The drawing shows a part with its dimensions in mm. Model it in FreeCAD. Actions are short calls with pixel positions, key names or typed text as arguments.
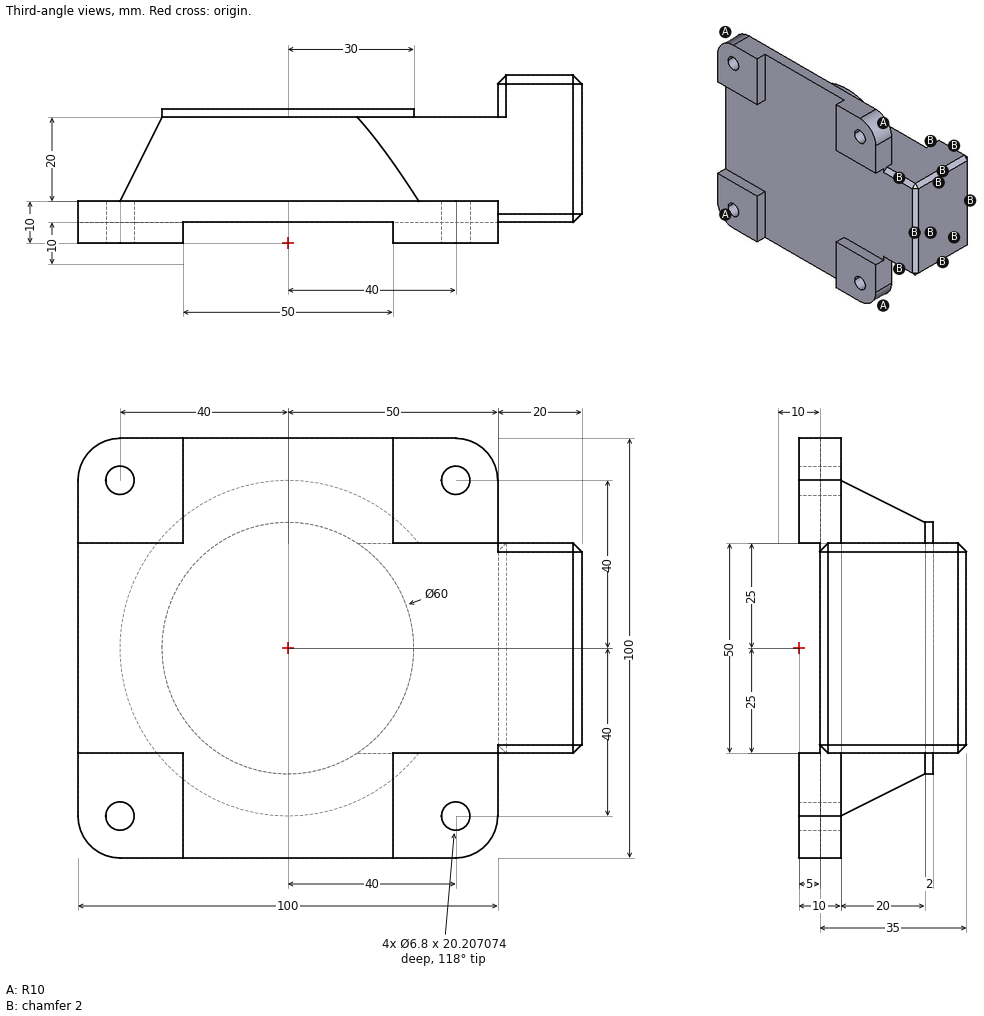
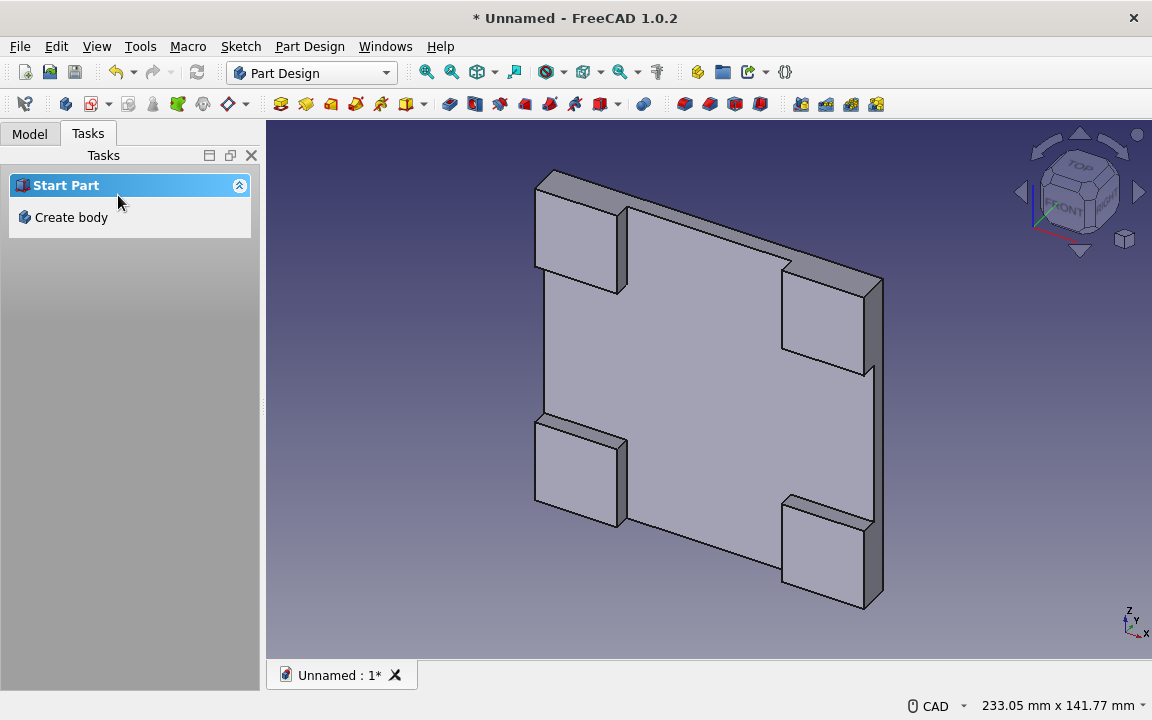
click(874, 287)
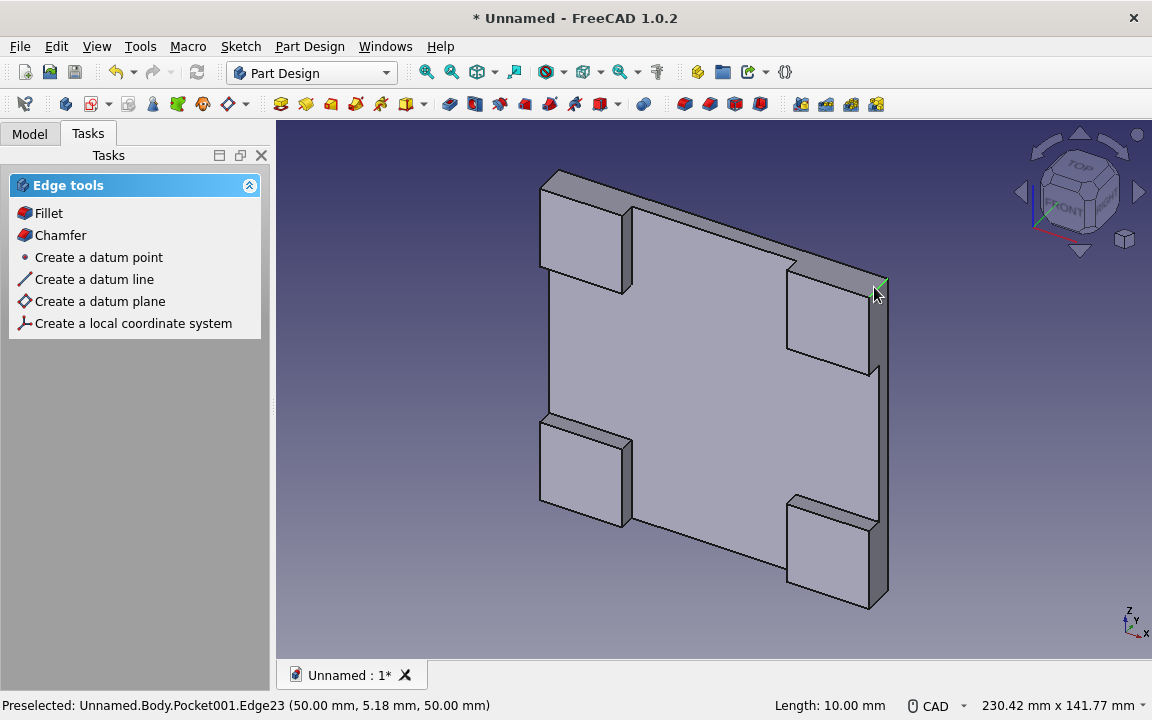
key(0)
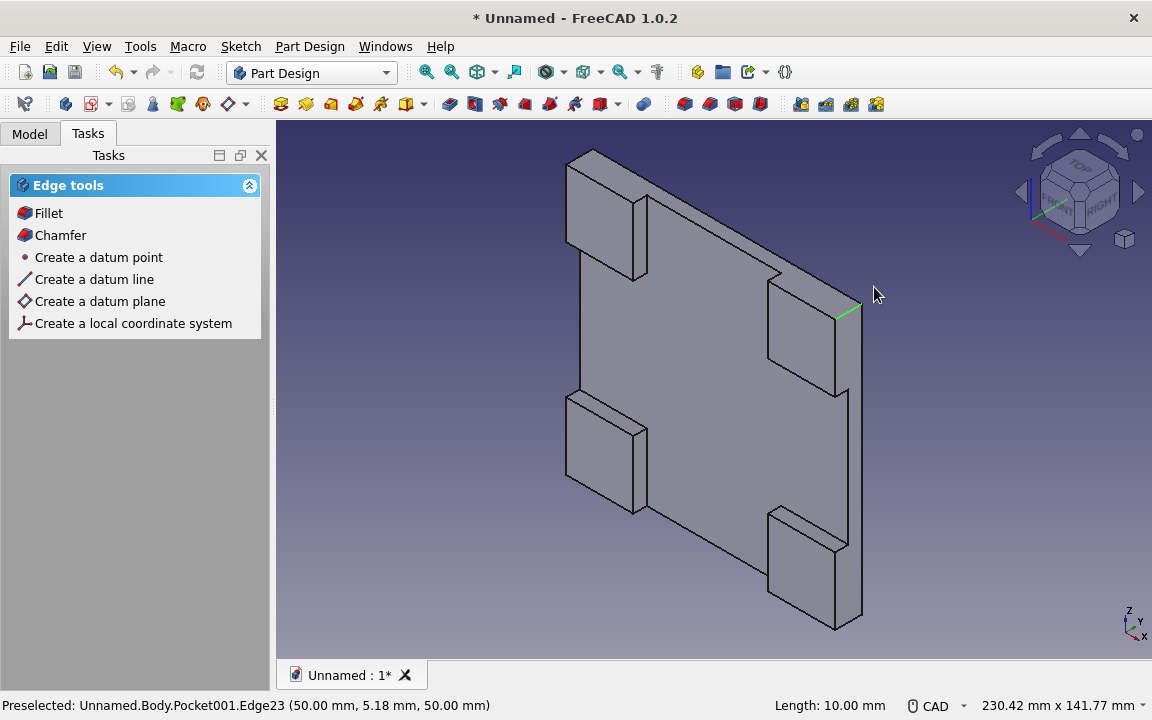
key(2)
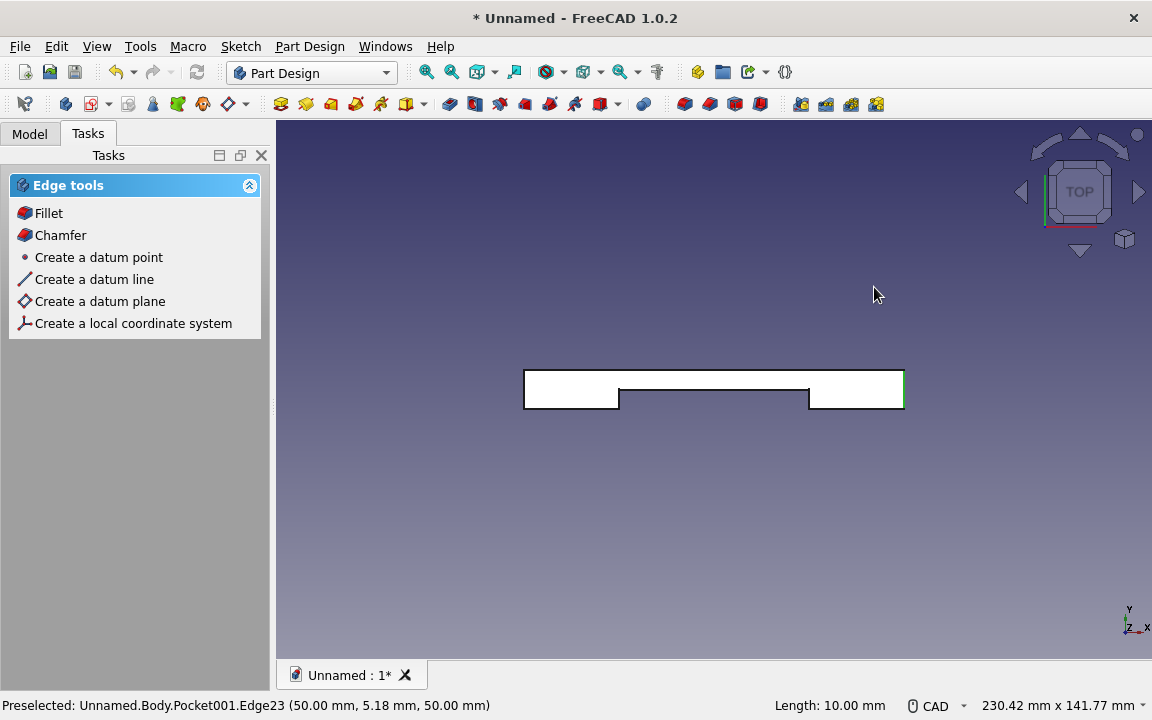
key(v)
key(f)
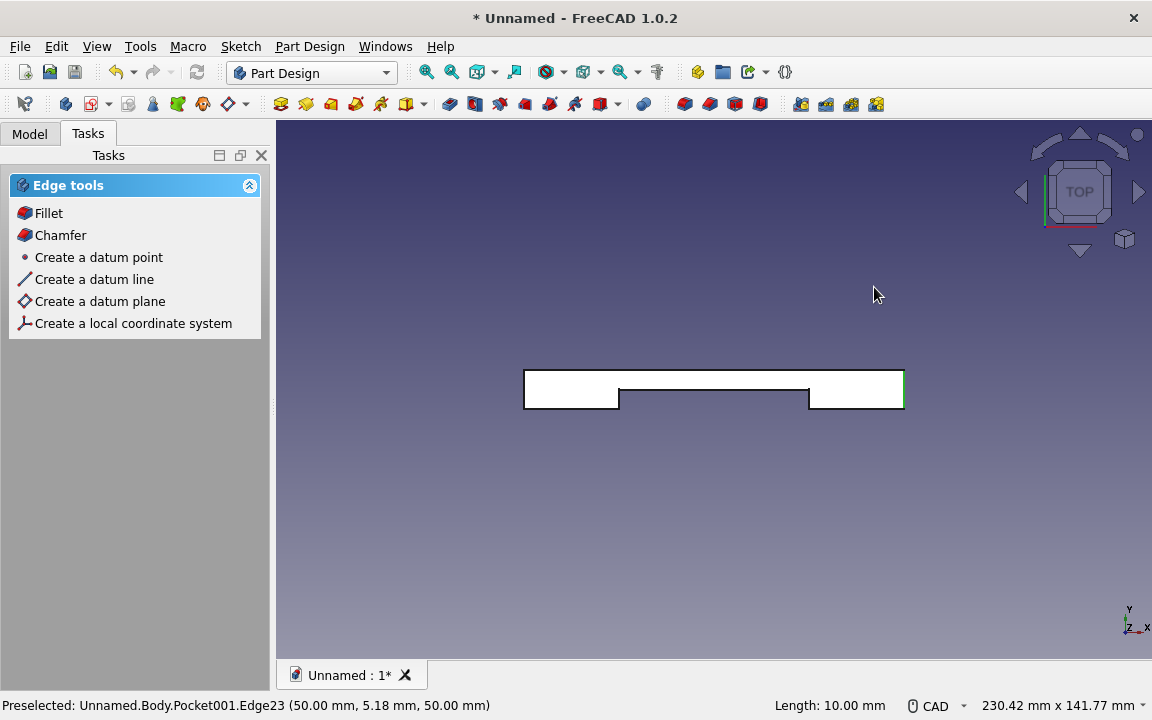
click(524, 388, ctrl)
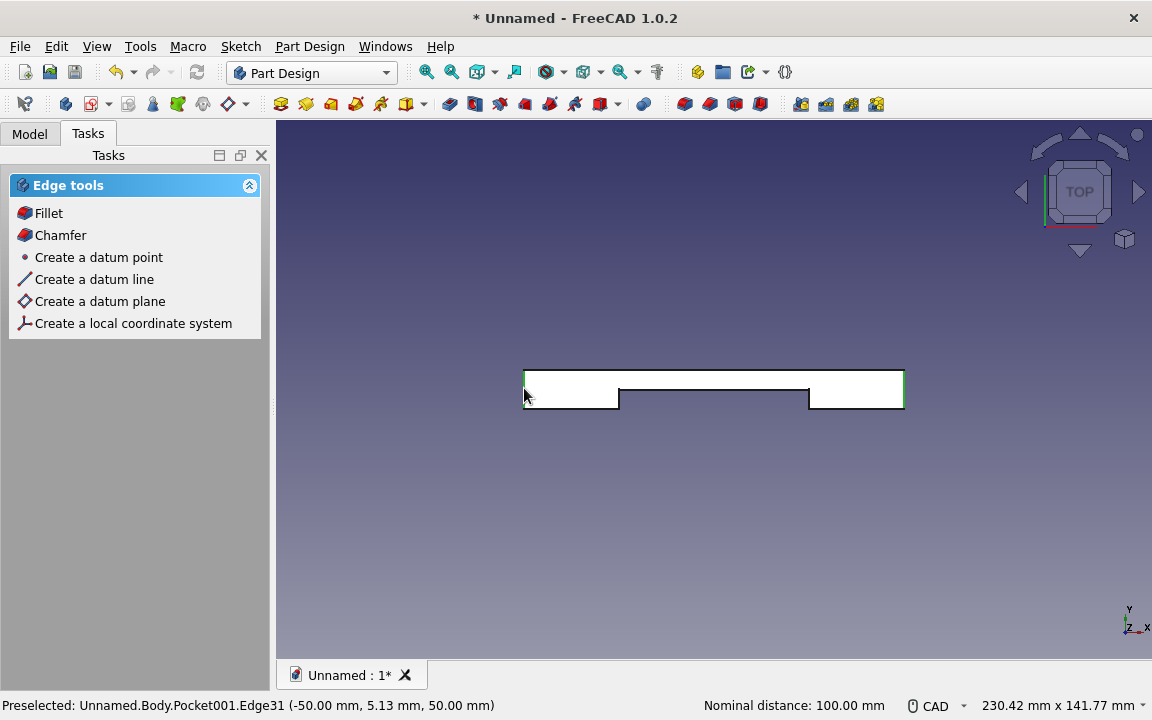
key(1)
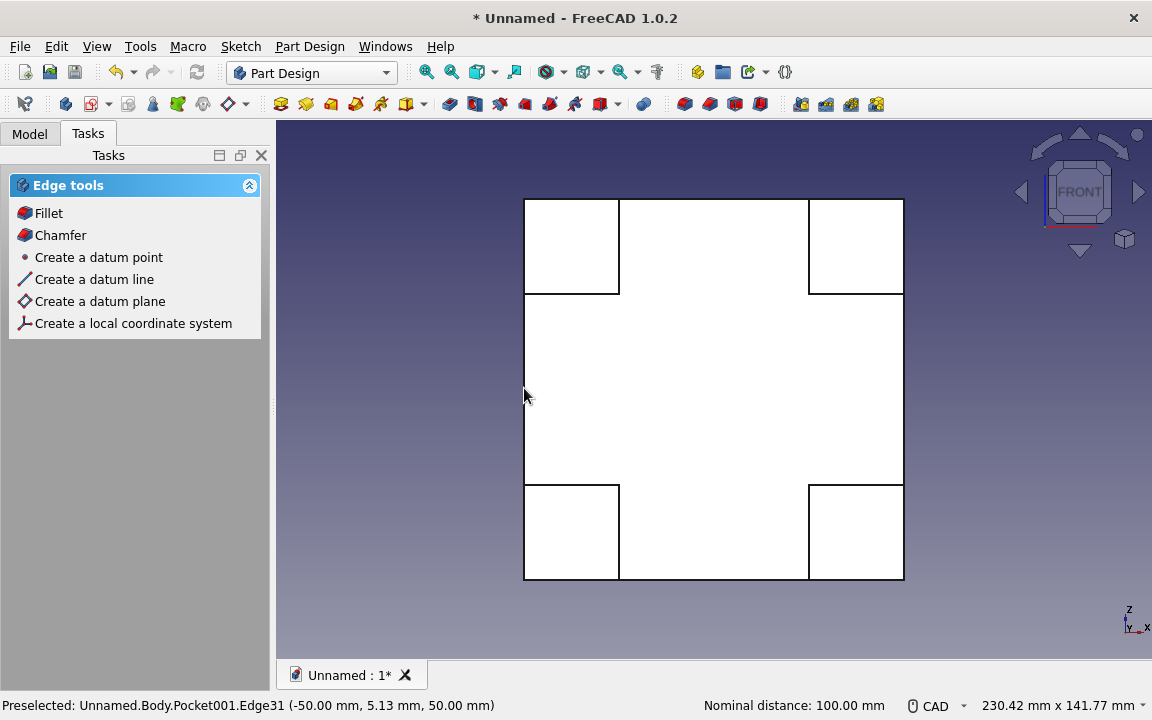
key(3)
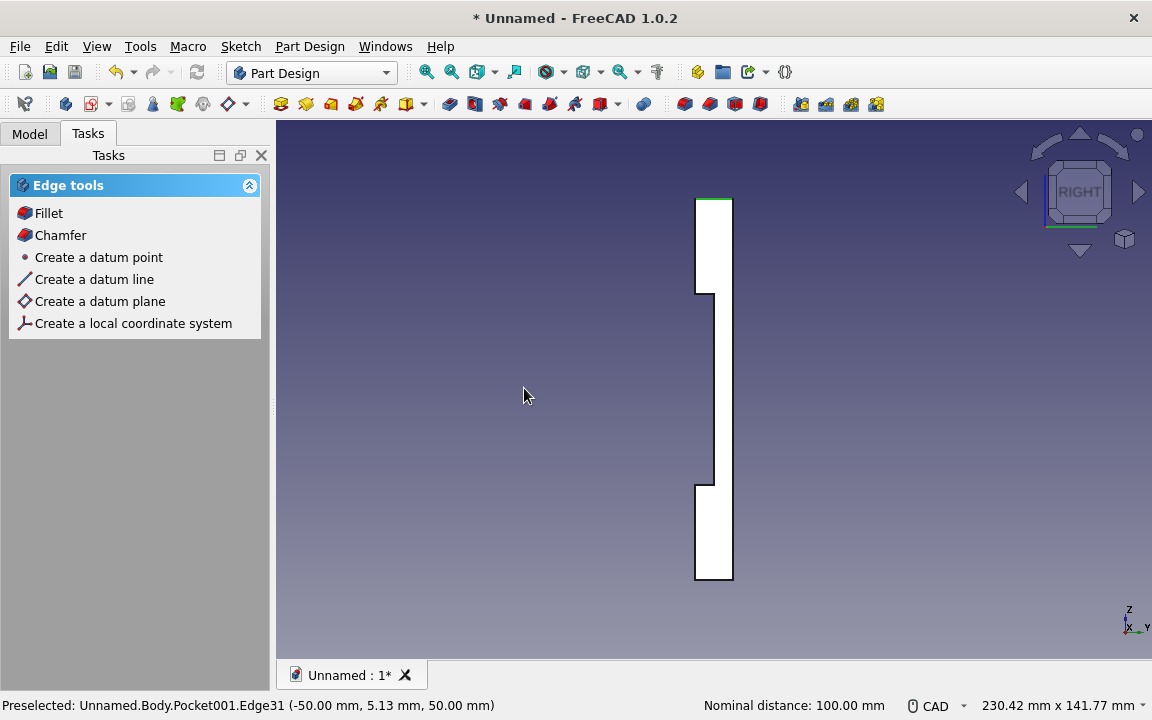
click(714, 579, ctrl)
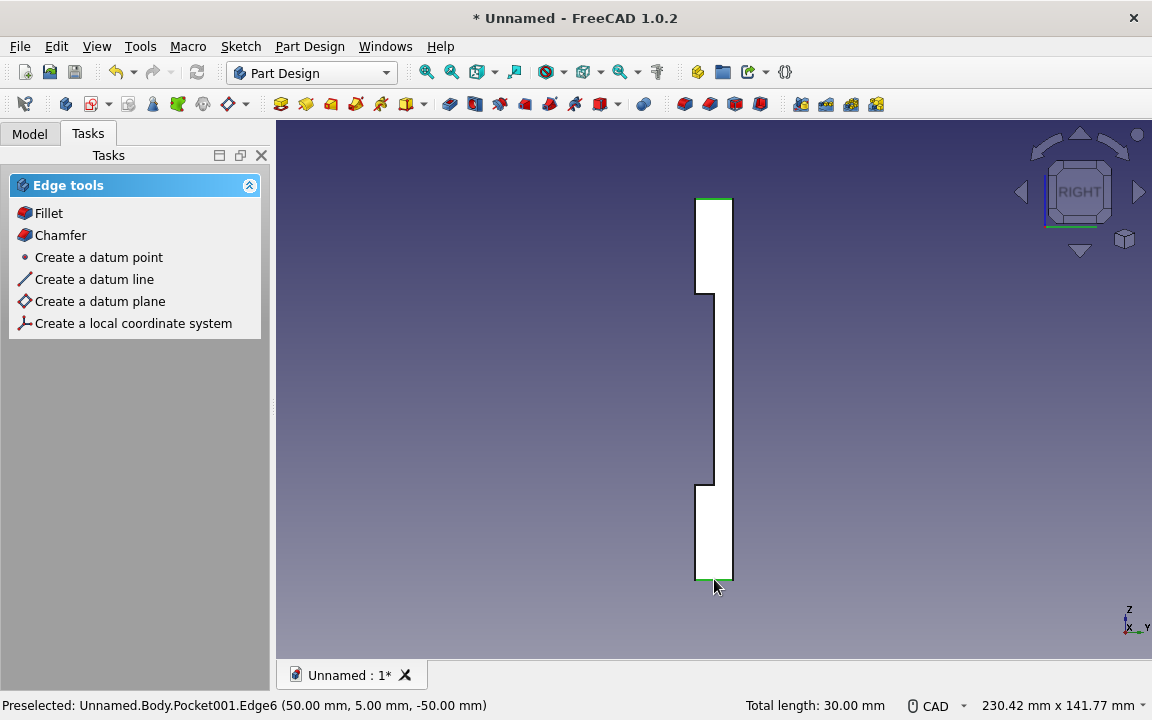
key(5)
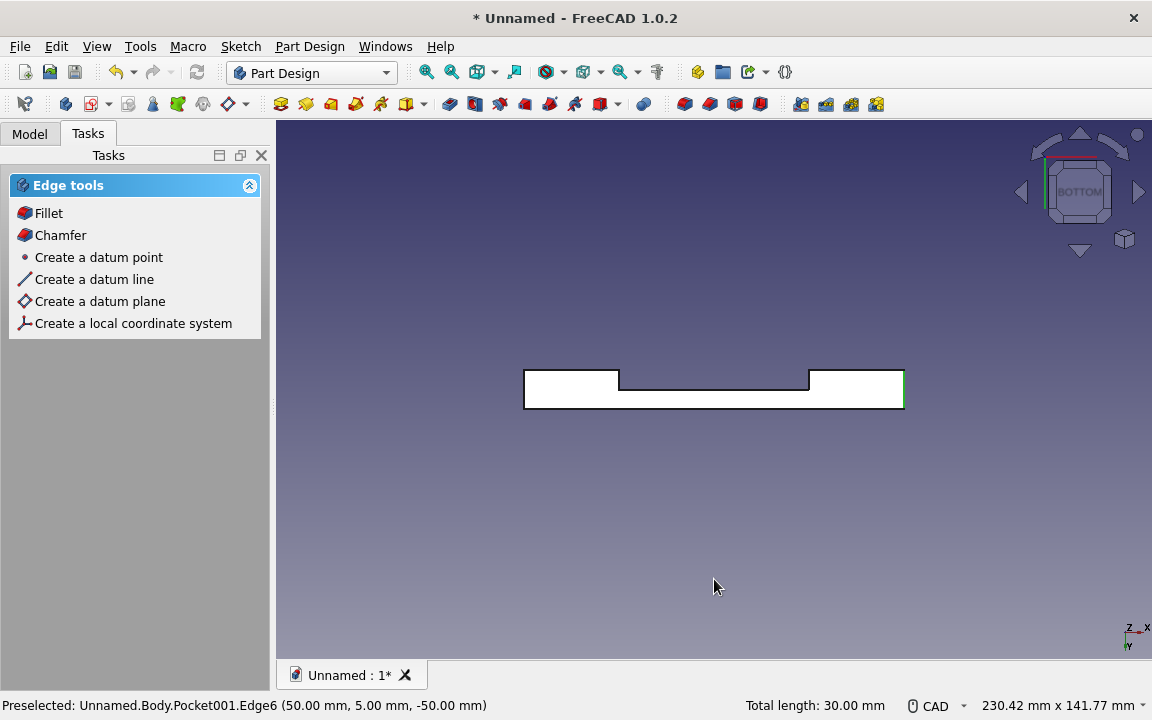
click(427, 72)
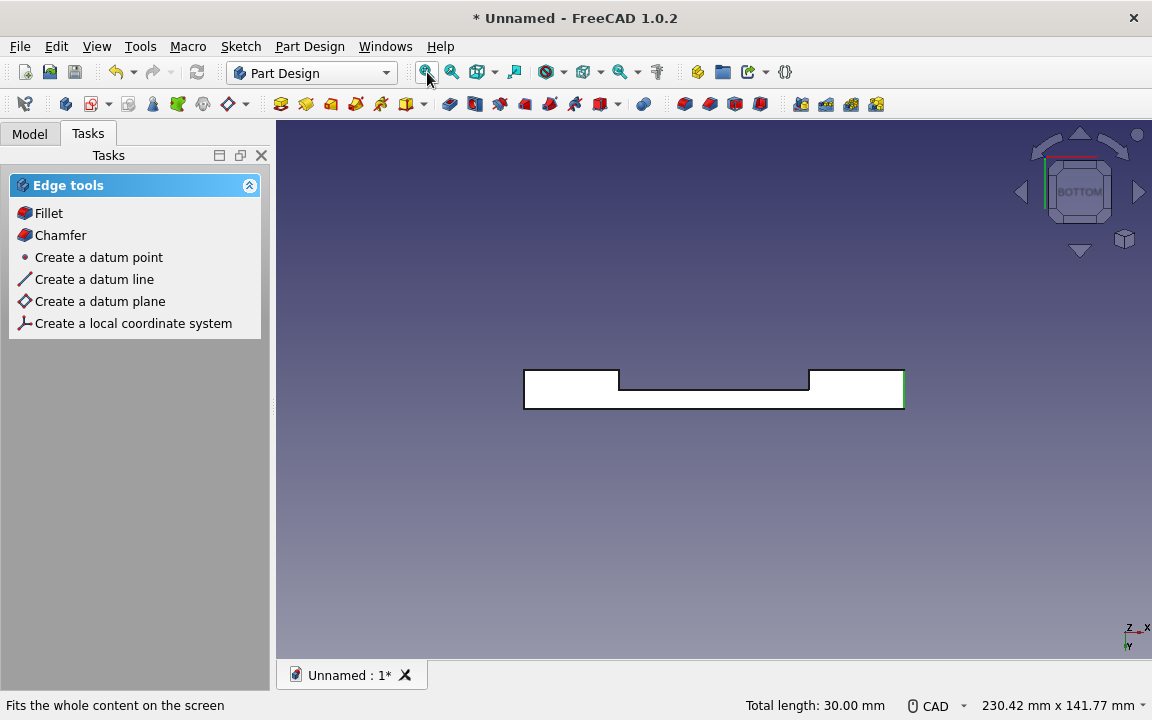
click(524, 388, ctrl)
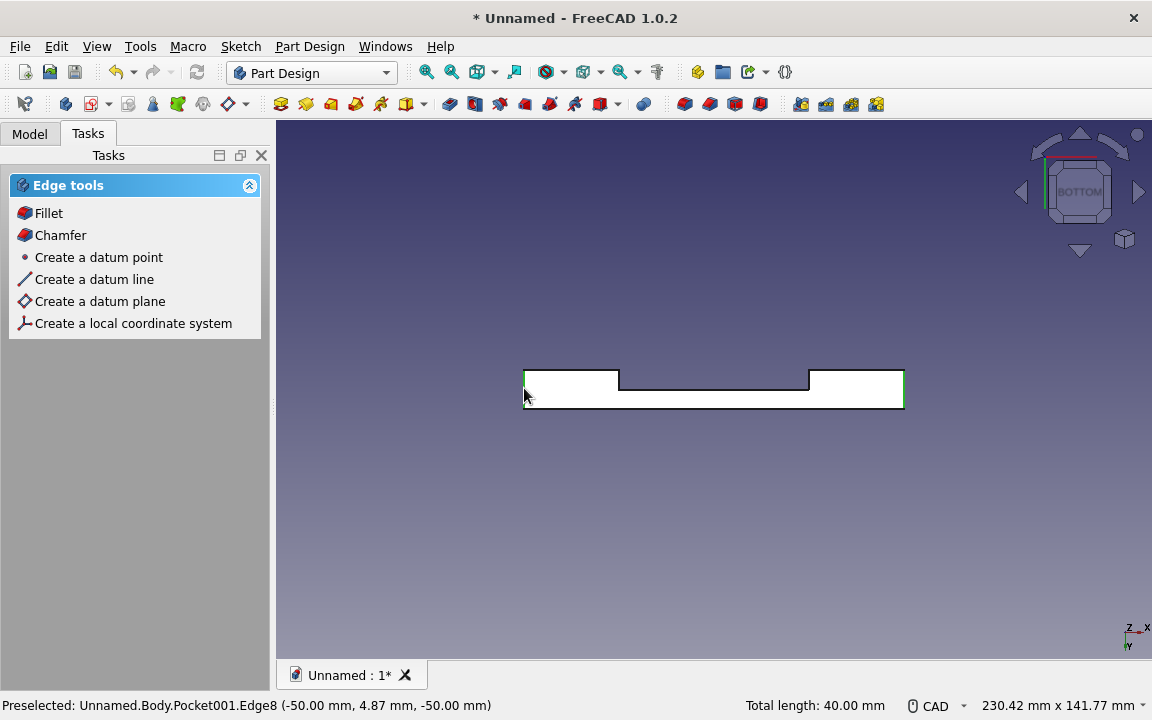
click(685, 104)